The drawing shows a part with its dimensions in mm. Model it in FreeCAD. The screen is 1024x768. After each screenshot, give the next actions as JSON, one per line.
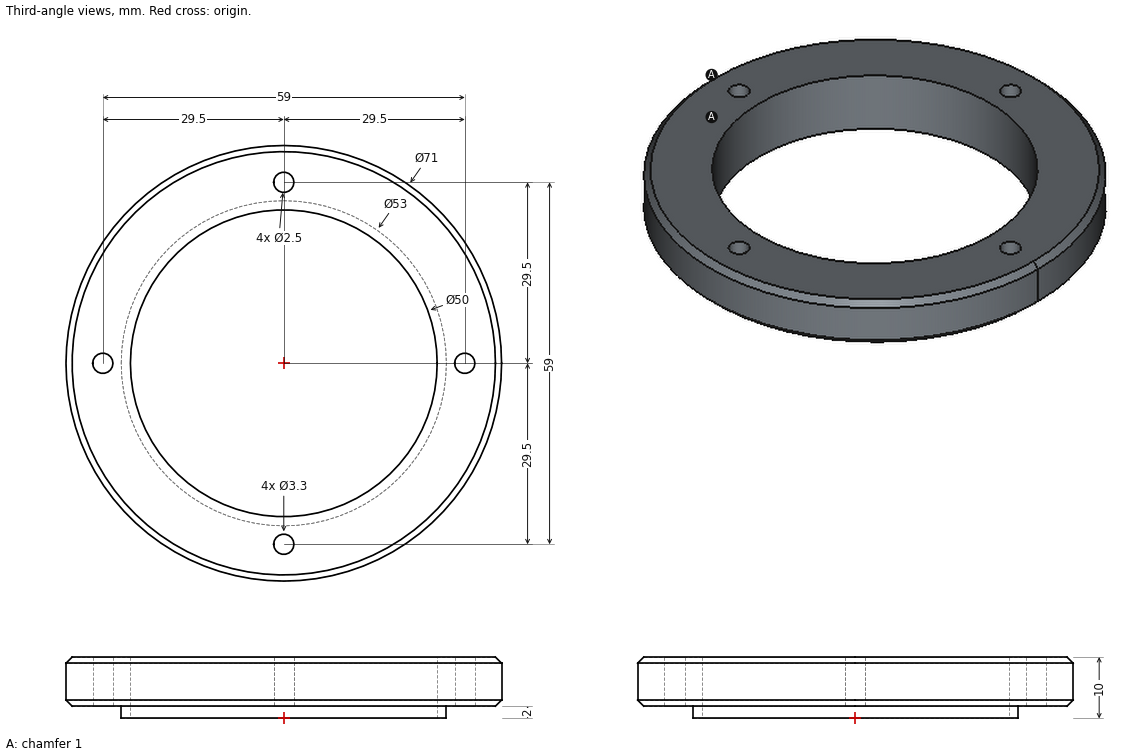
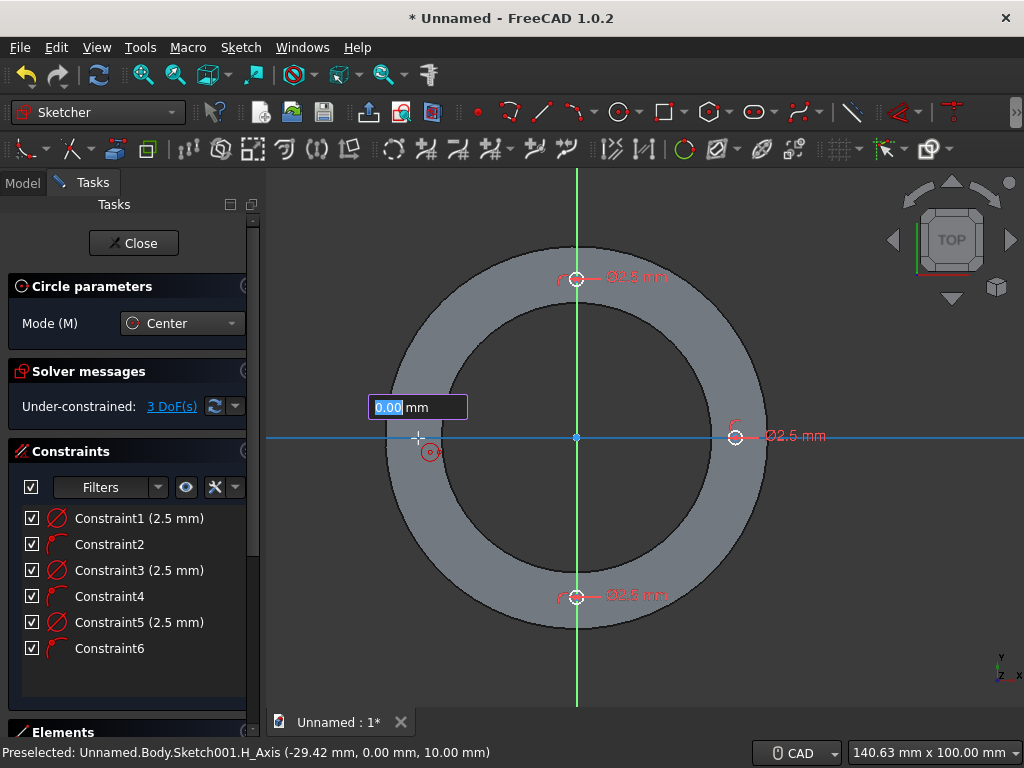
{"action": "scroll", "coordinate": [415, 444], "scroll_direction": "up", "scroll_amount": 5}
{"action": "mouse_move", "coordinate": [415, 443]}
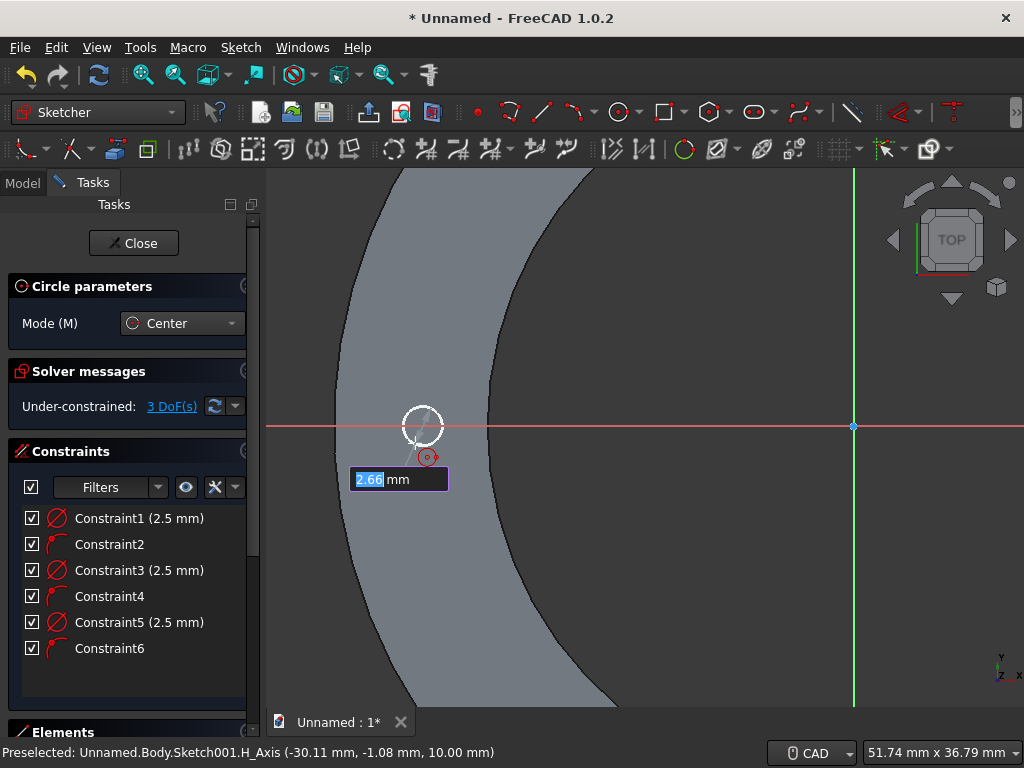
{"action": "type", "text": "2.5"}
{"action": "key", "text": "Return"}
{"action": "key", "text": "Escape"}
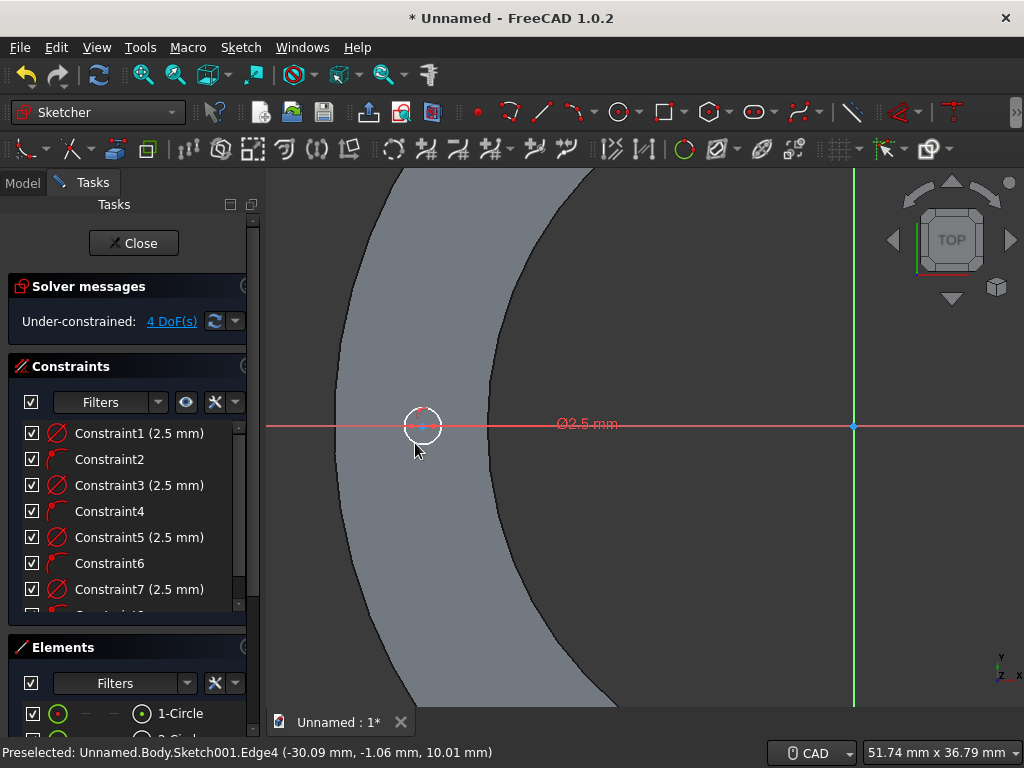
{"action": "scroll", "coordinate": [415, 444], "scroll_direction": "down", "scroll_amount": 5}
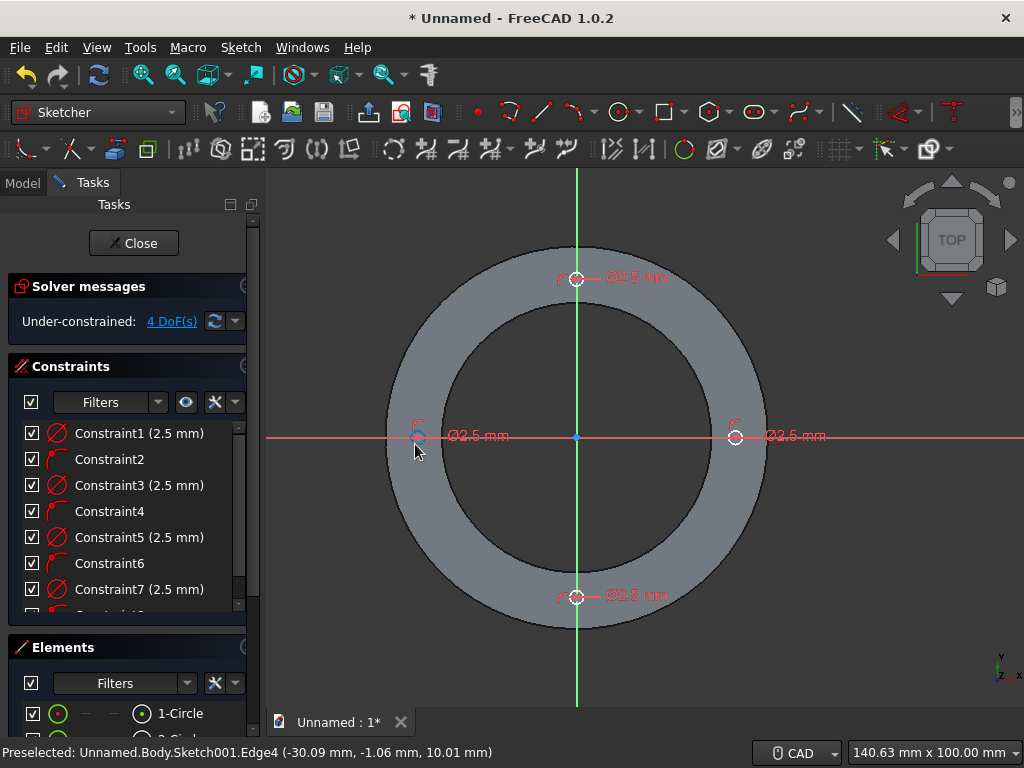
{"action": "left_click", "coordinate": [577, 279]}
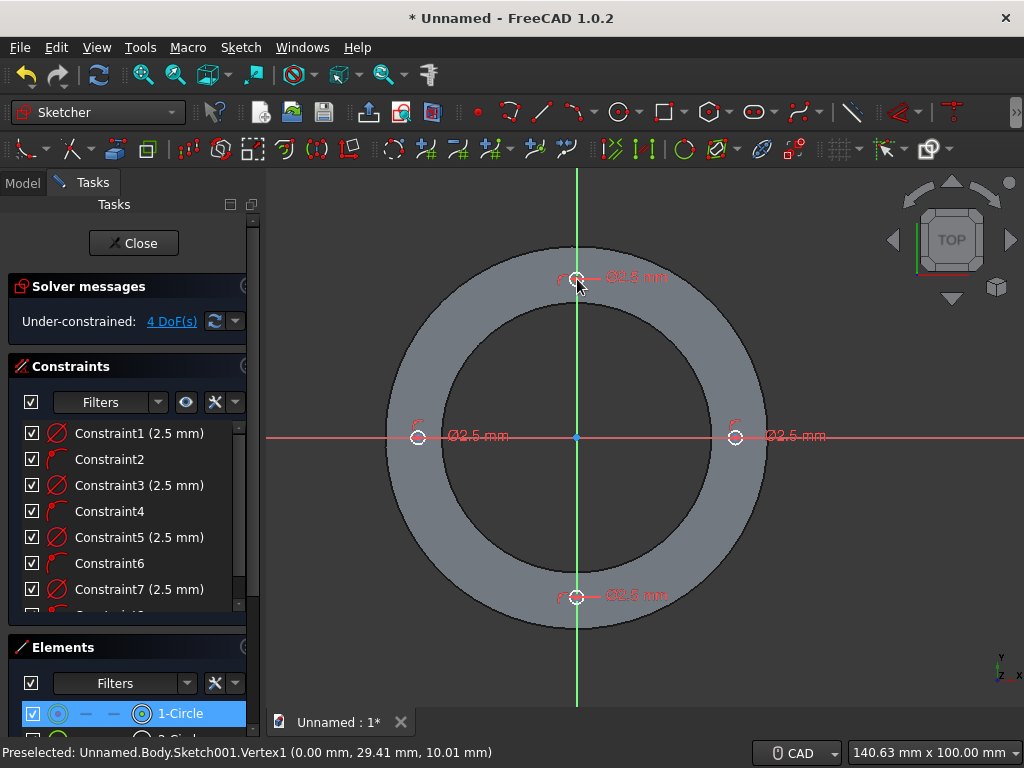
{"action": "left_click", "coordinate": [577, 597]}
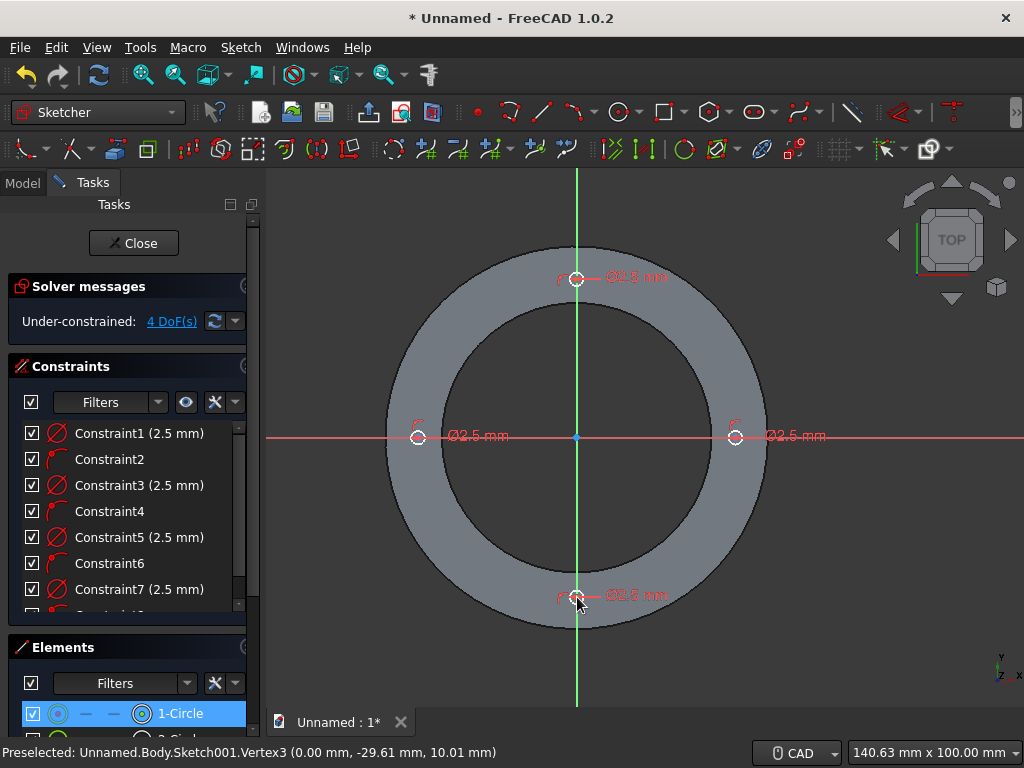
{"action": "key", "text": "i"}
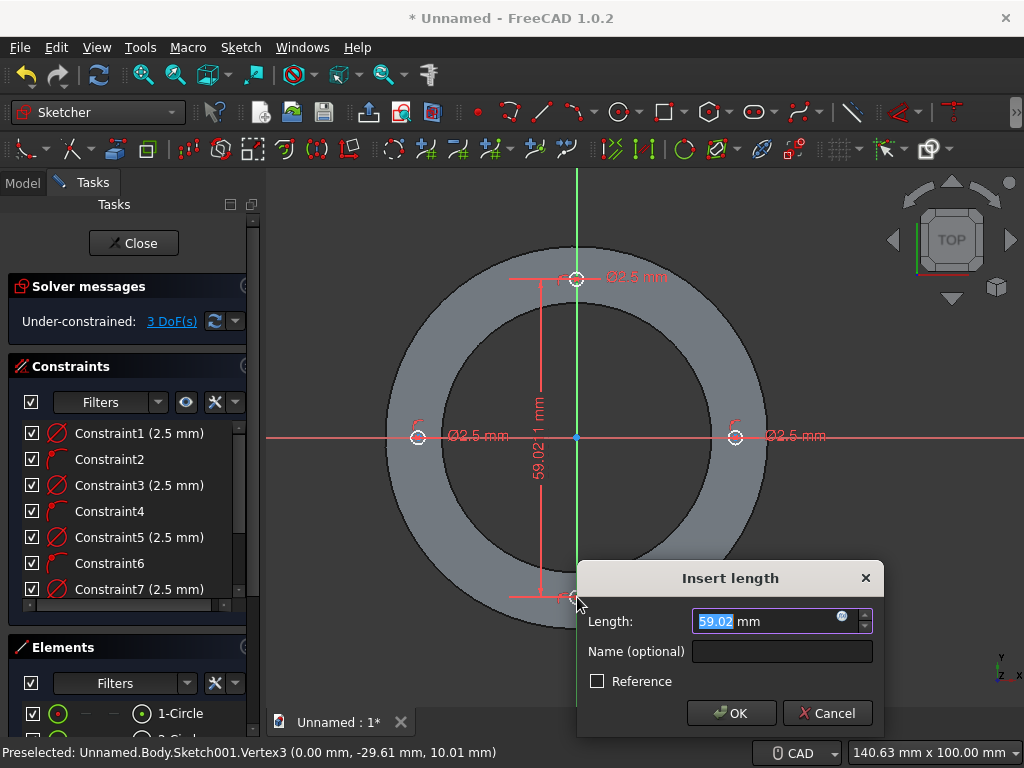
{"action": "type", "text": "59"}
{"action": "key", "text": "Return"}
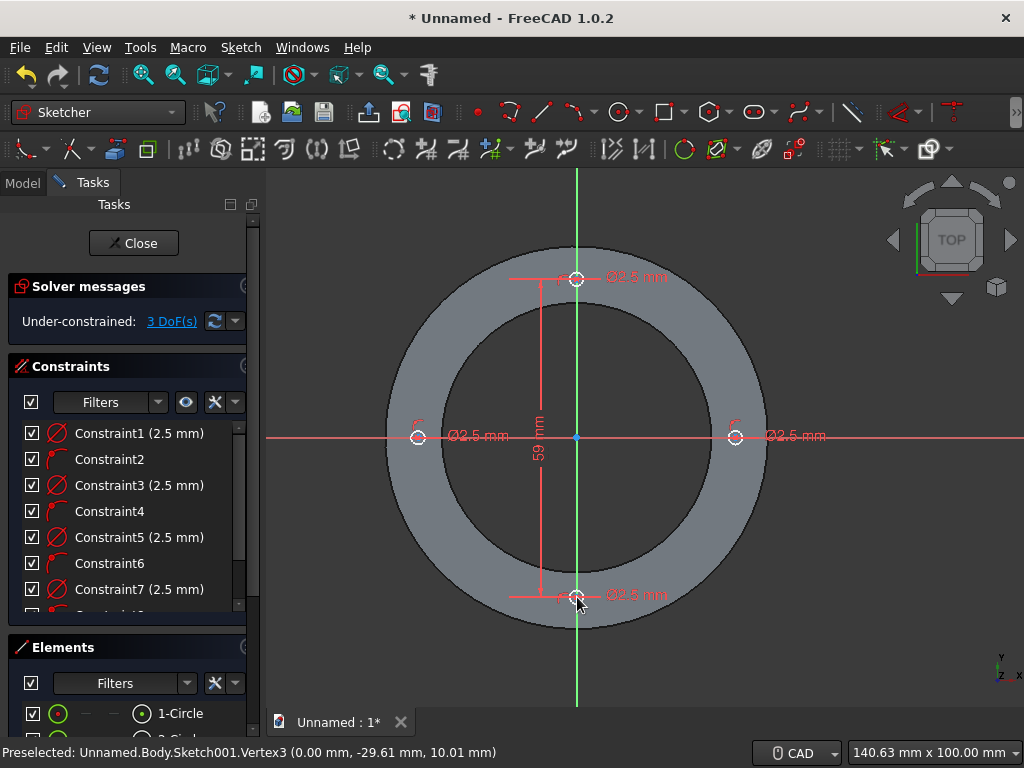
{"action": "left_click", "coordinate": [735, 438]}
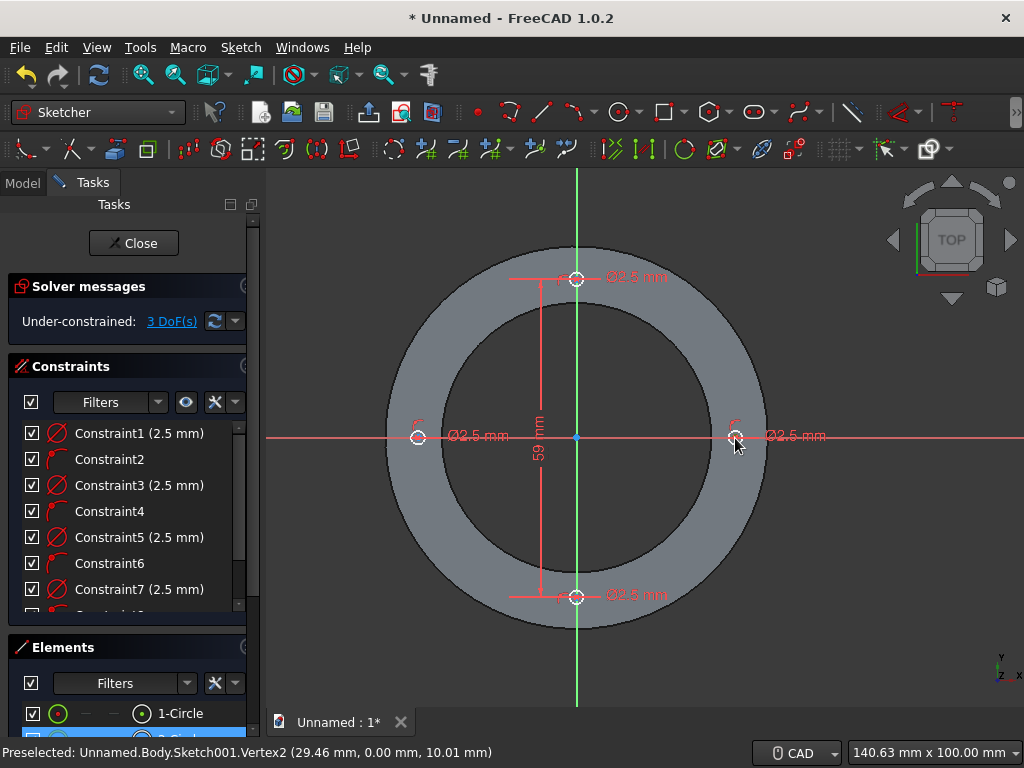
{"action": "left_click", "coordinate": [418, 438]}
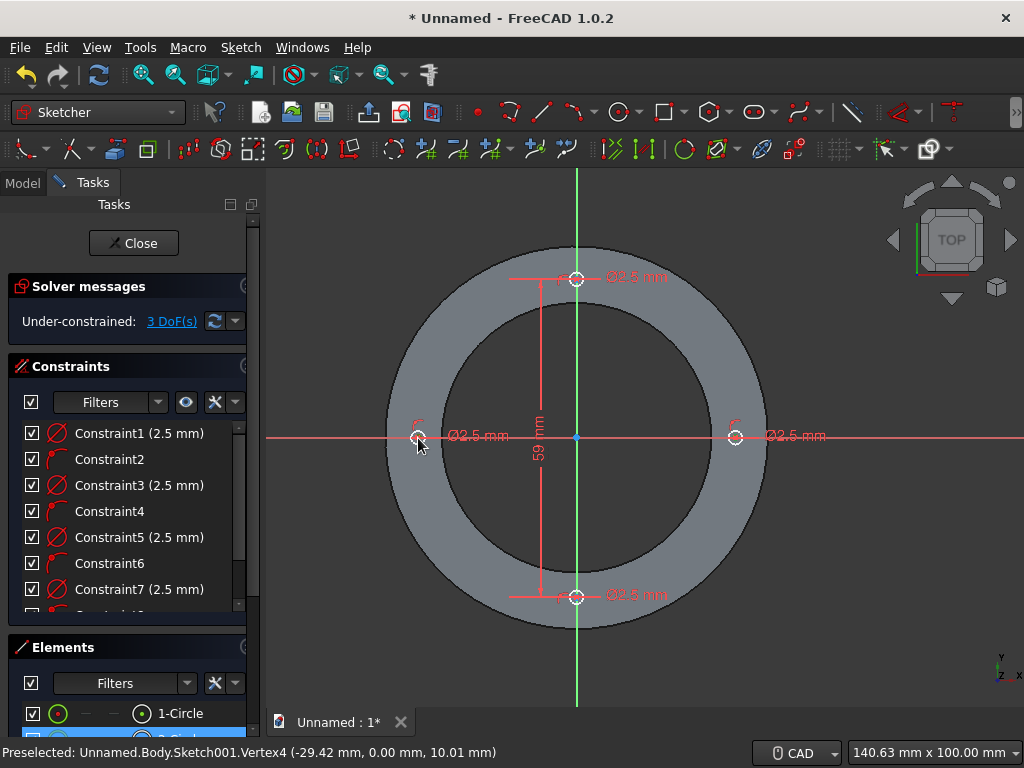
{"action": "key", "text": "l"}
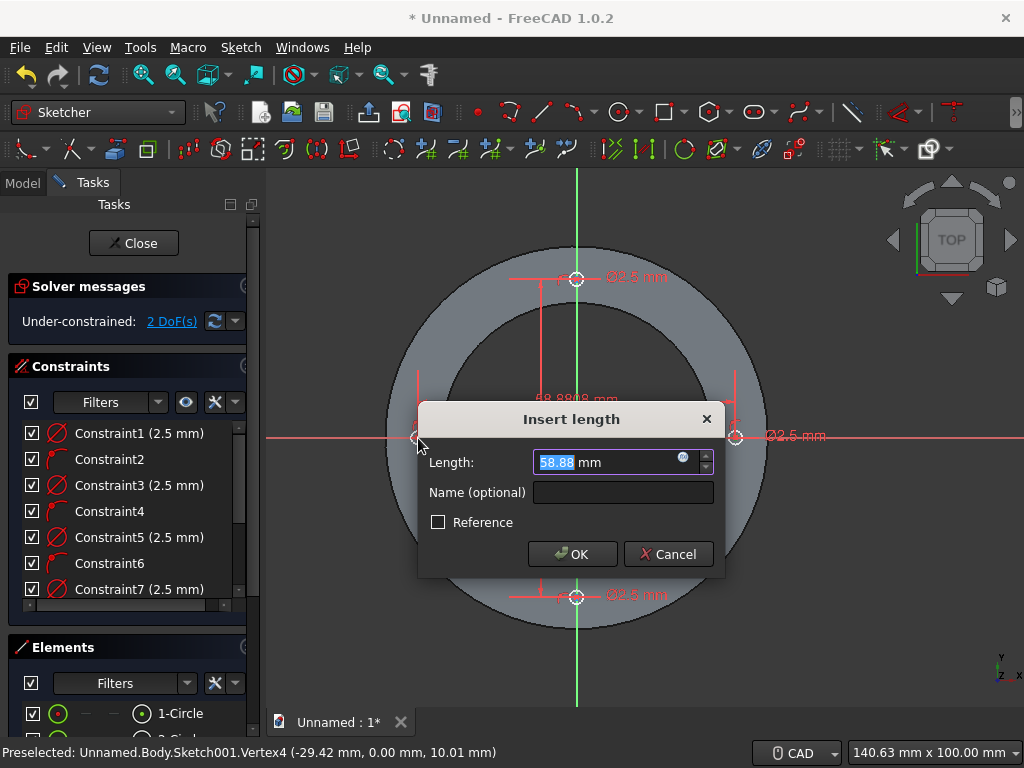
{"action": "type", "text": "59"}
{"action": "key", "text": "Return"}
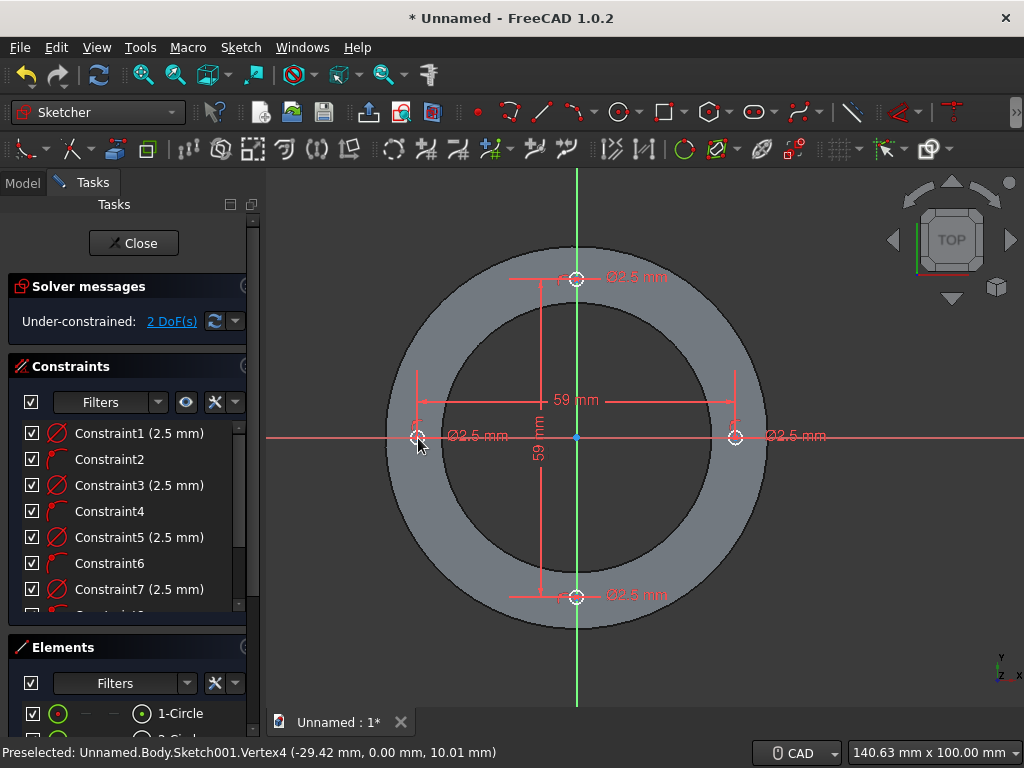
{"action": "left_click", "coordinate": [577, 279]}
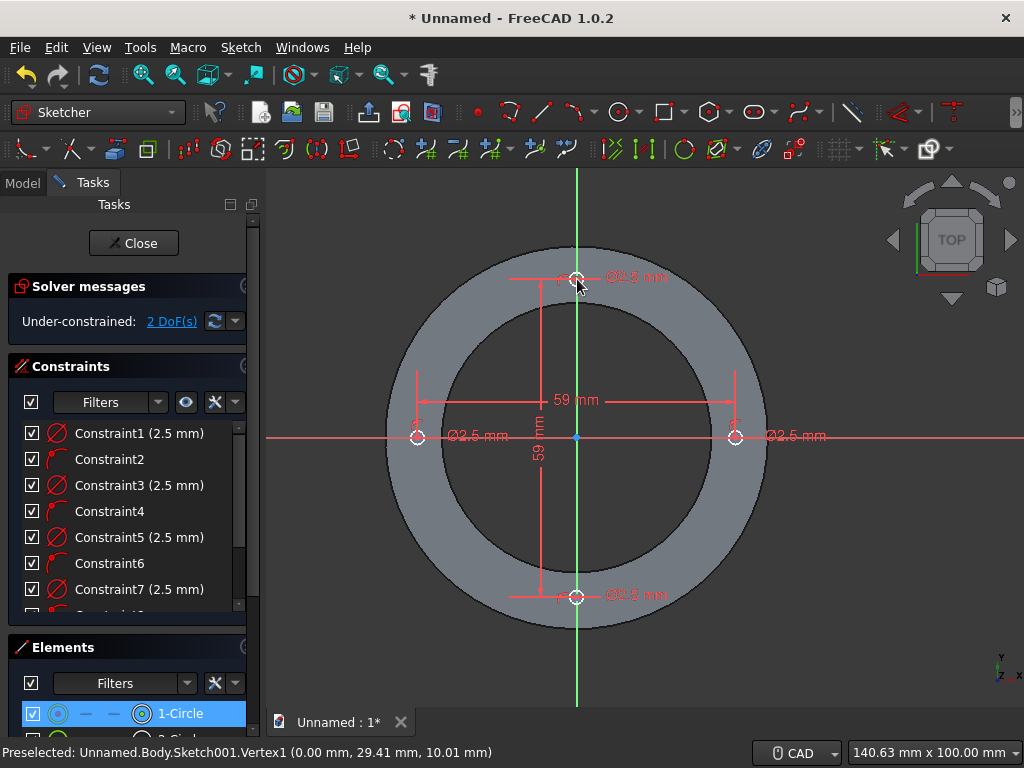
{"action": "key", "text": "i"}